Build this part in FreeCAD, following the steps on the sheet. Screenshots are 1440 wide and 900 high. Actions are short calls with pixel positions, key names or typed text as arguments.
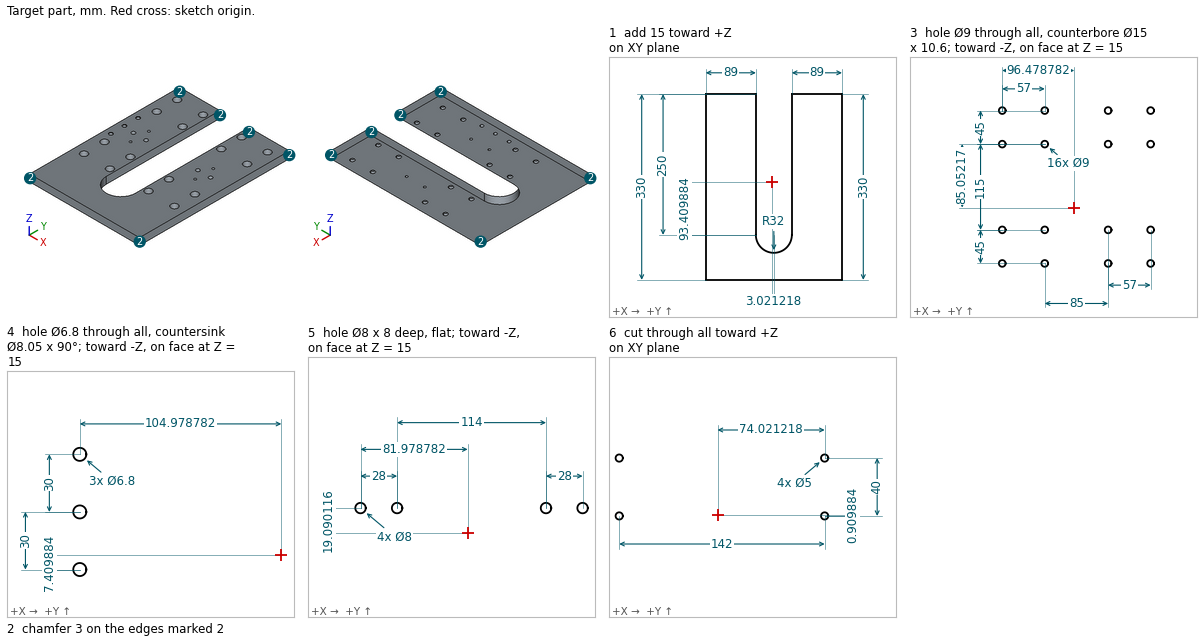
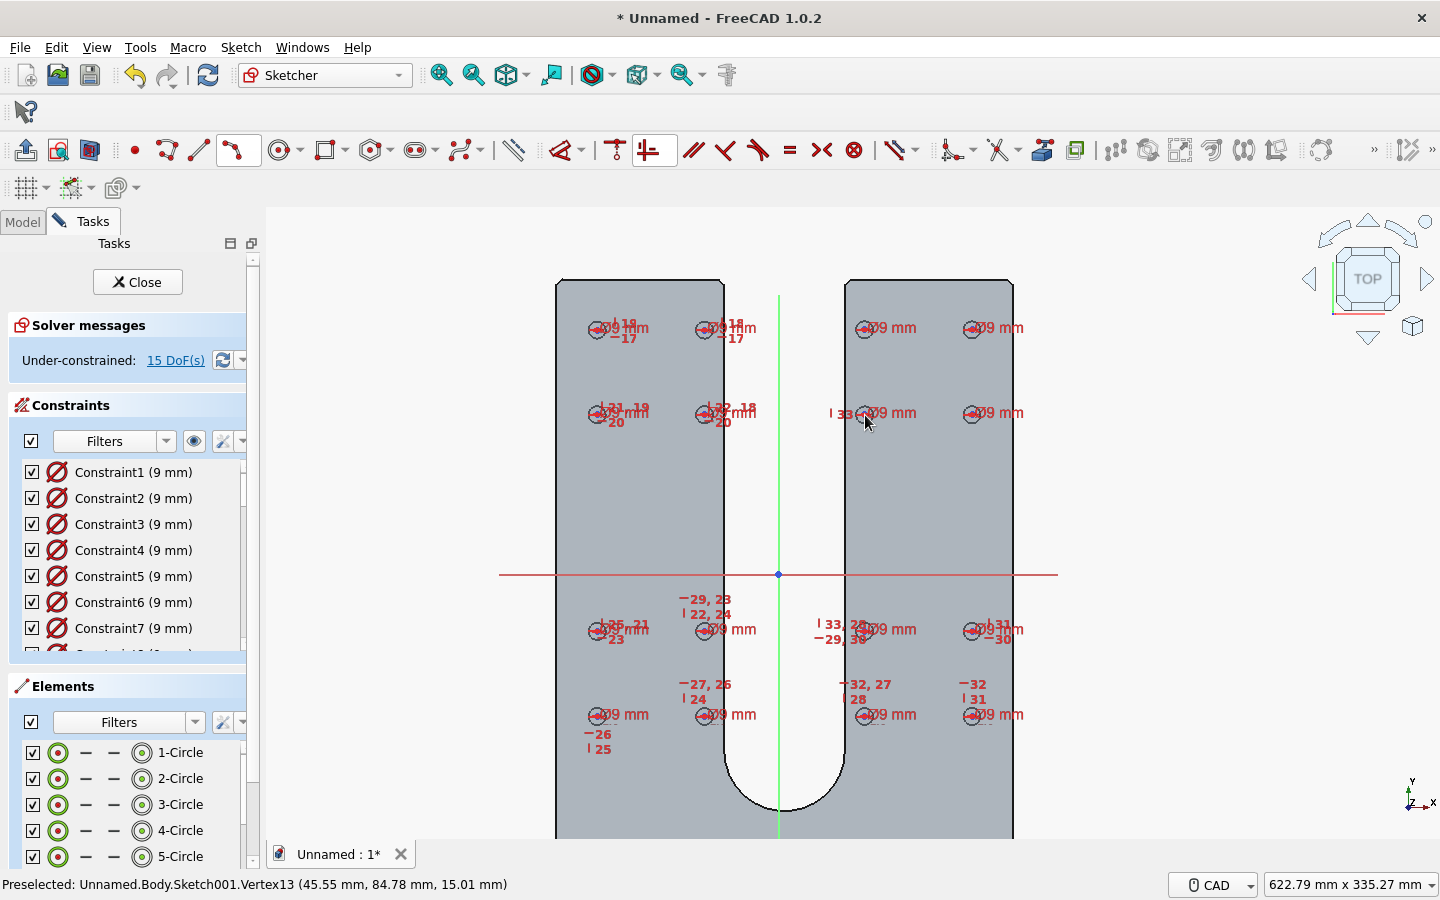
click(705, 415)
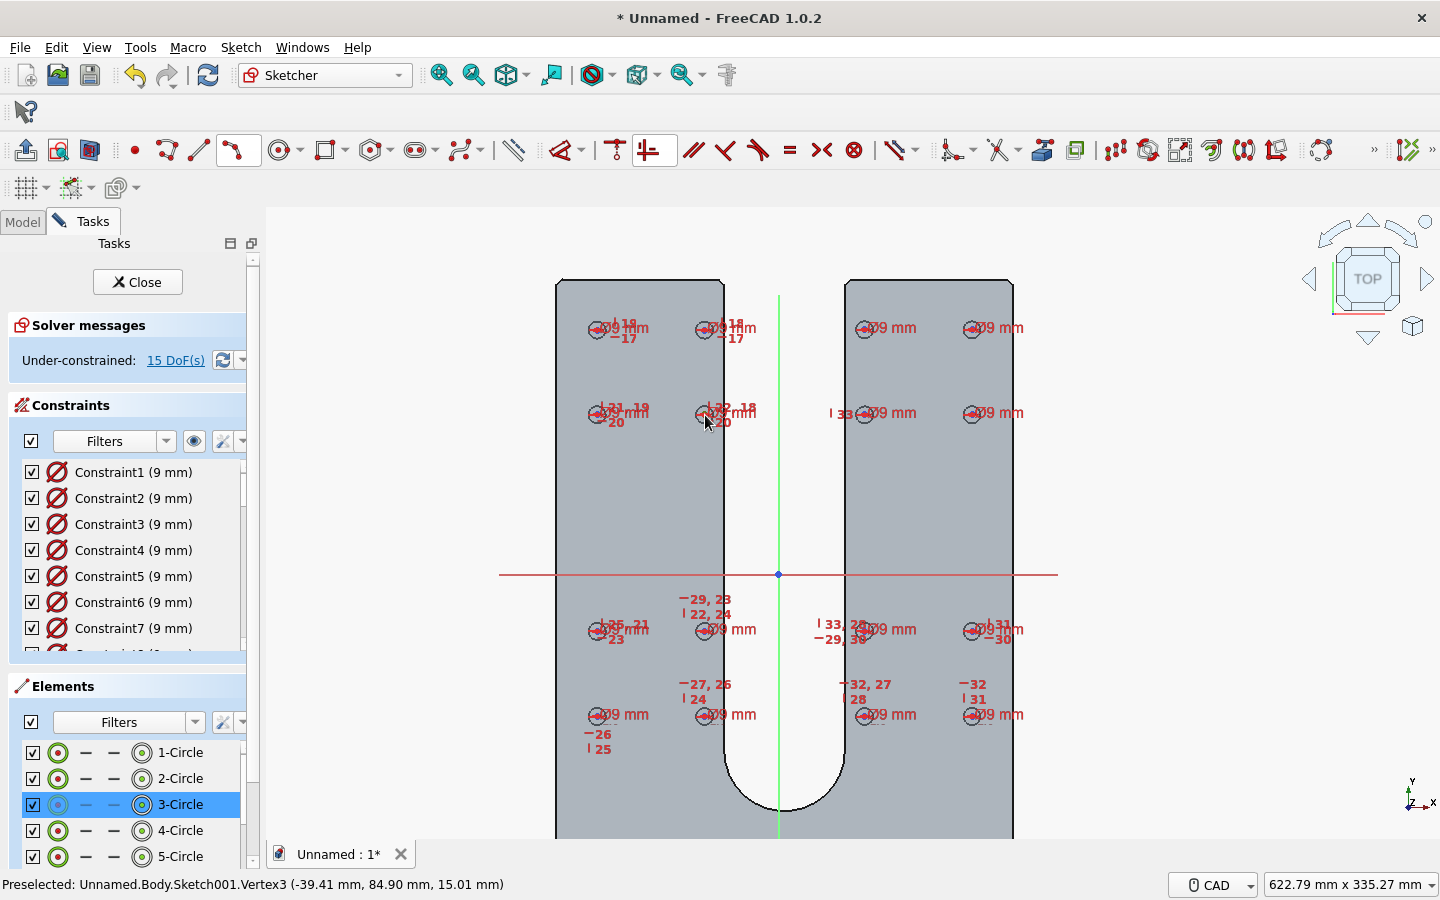
click(865, 415)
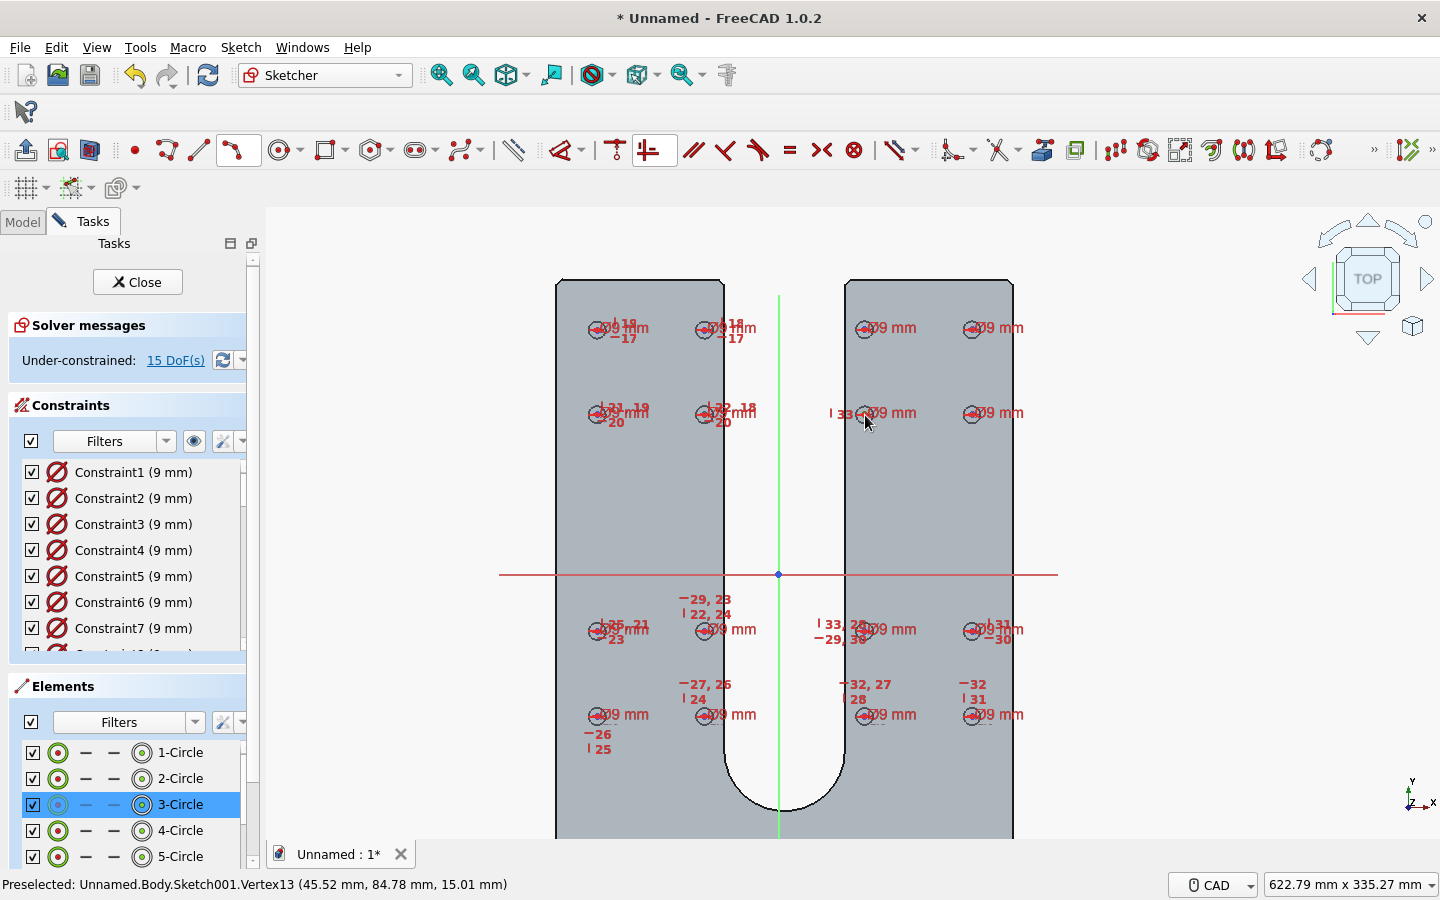
key(h)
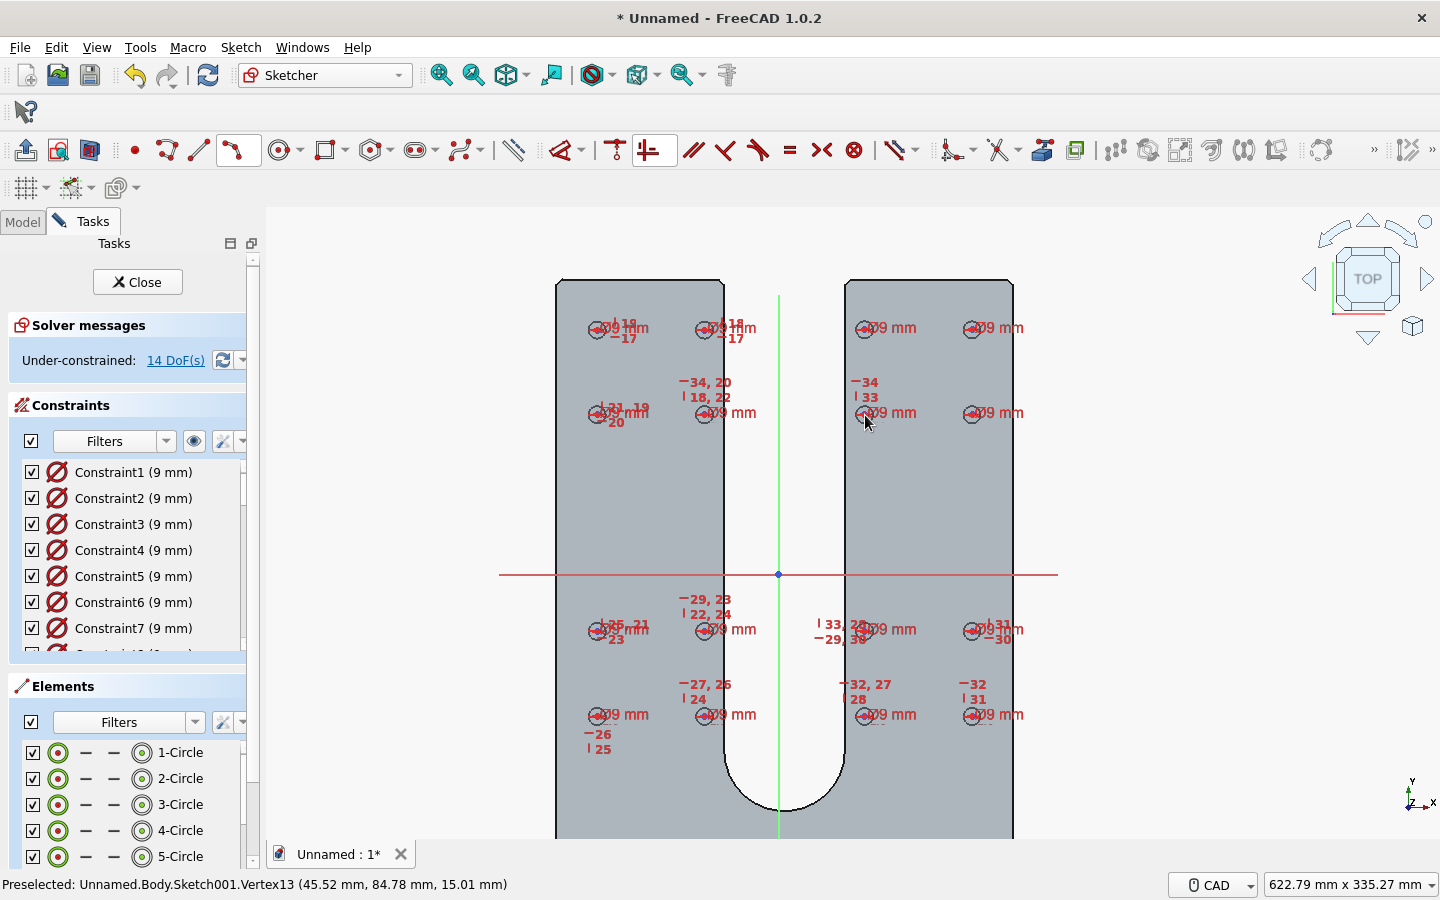
click(865, 415)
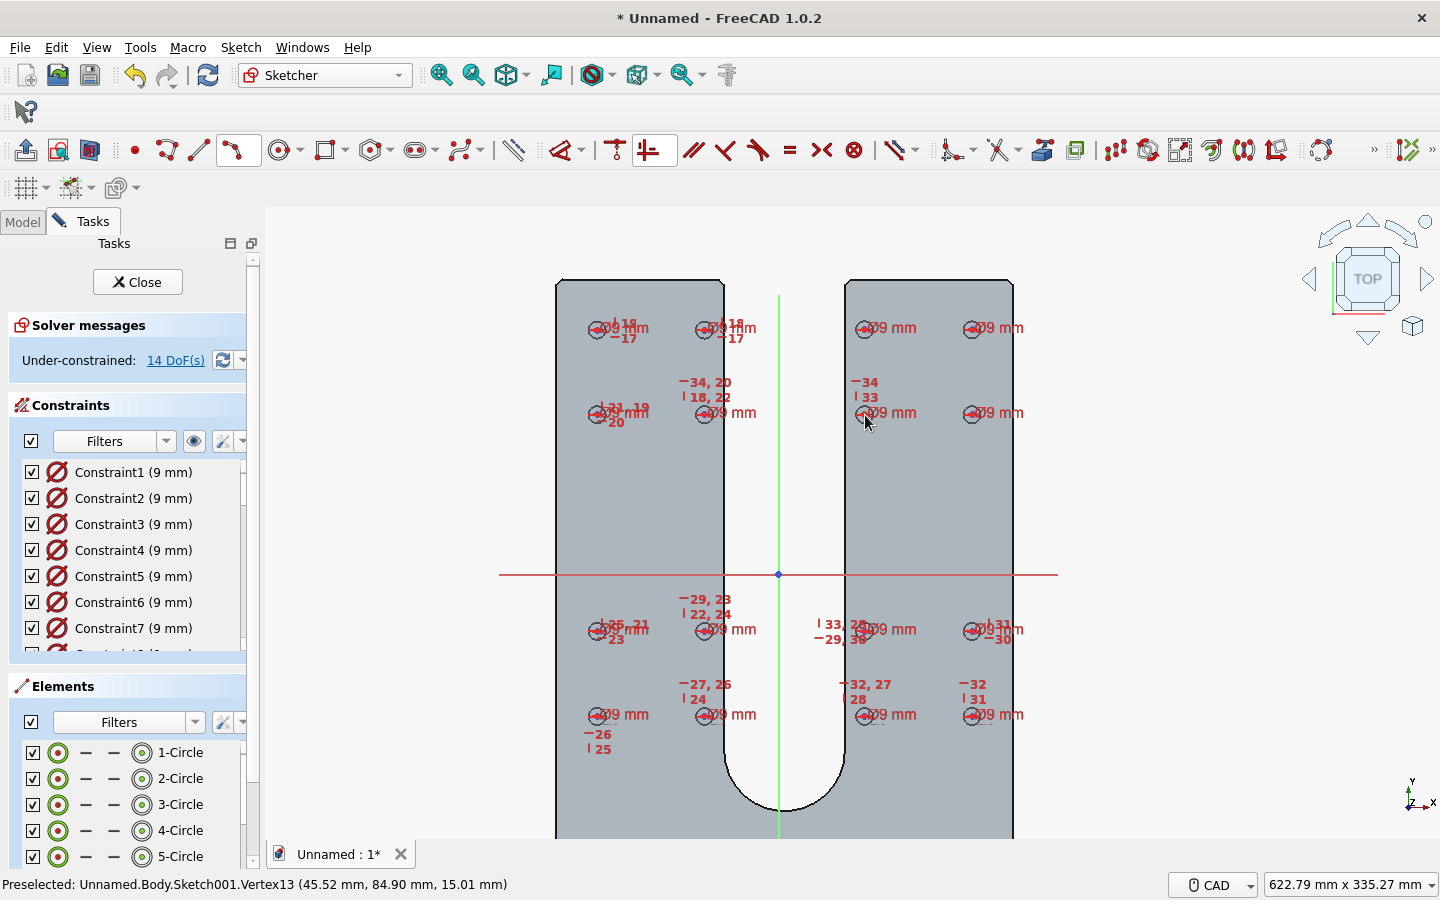
click(865, 330)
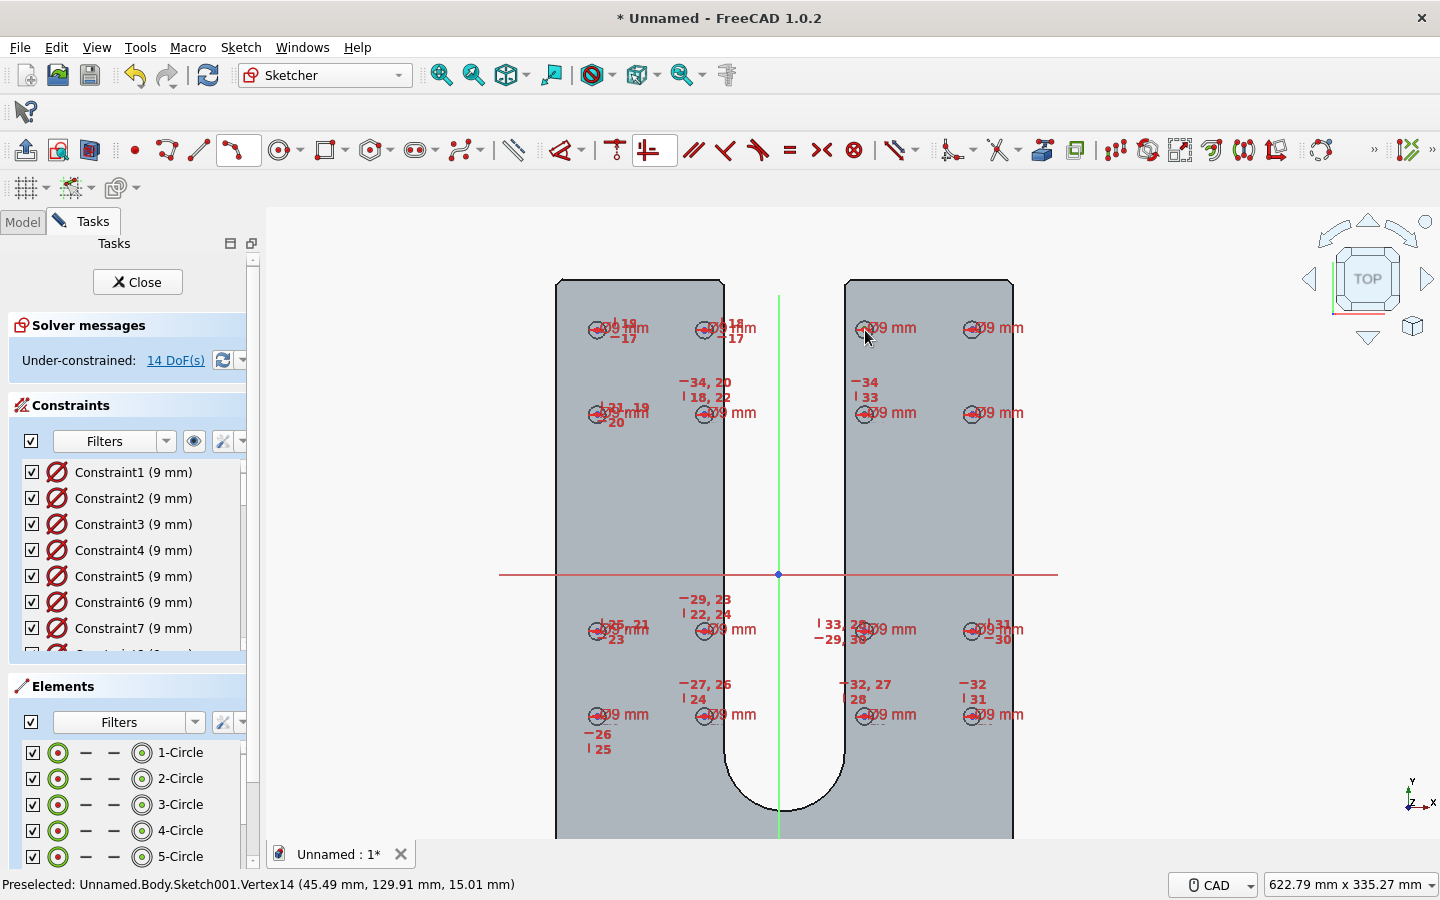
key(v)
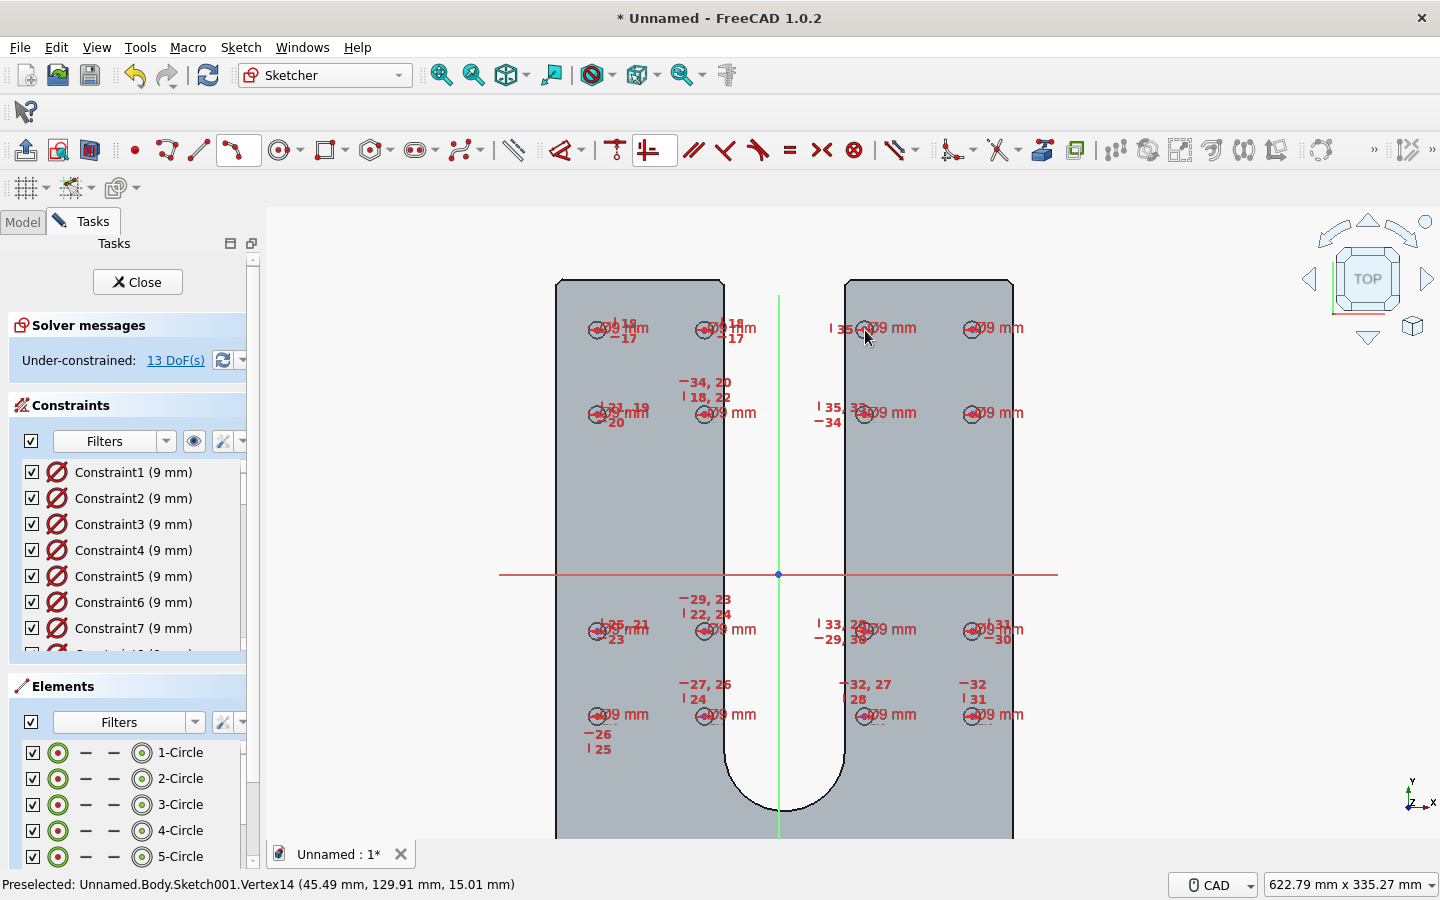
click(705, 330)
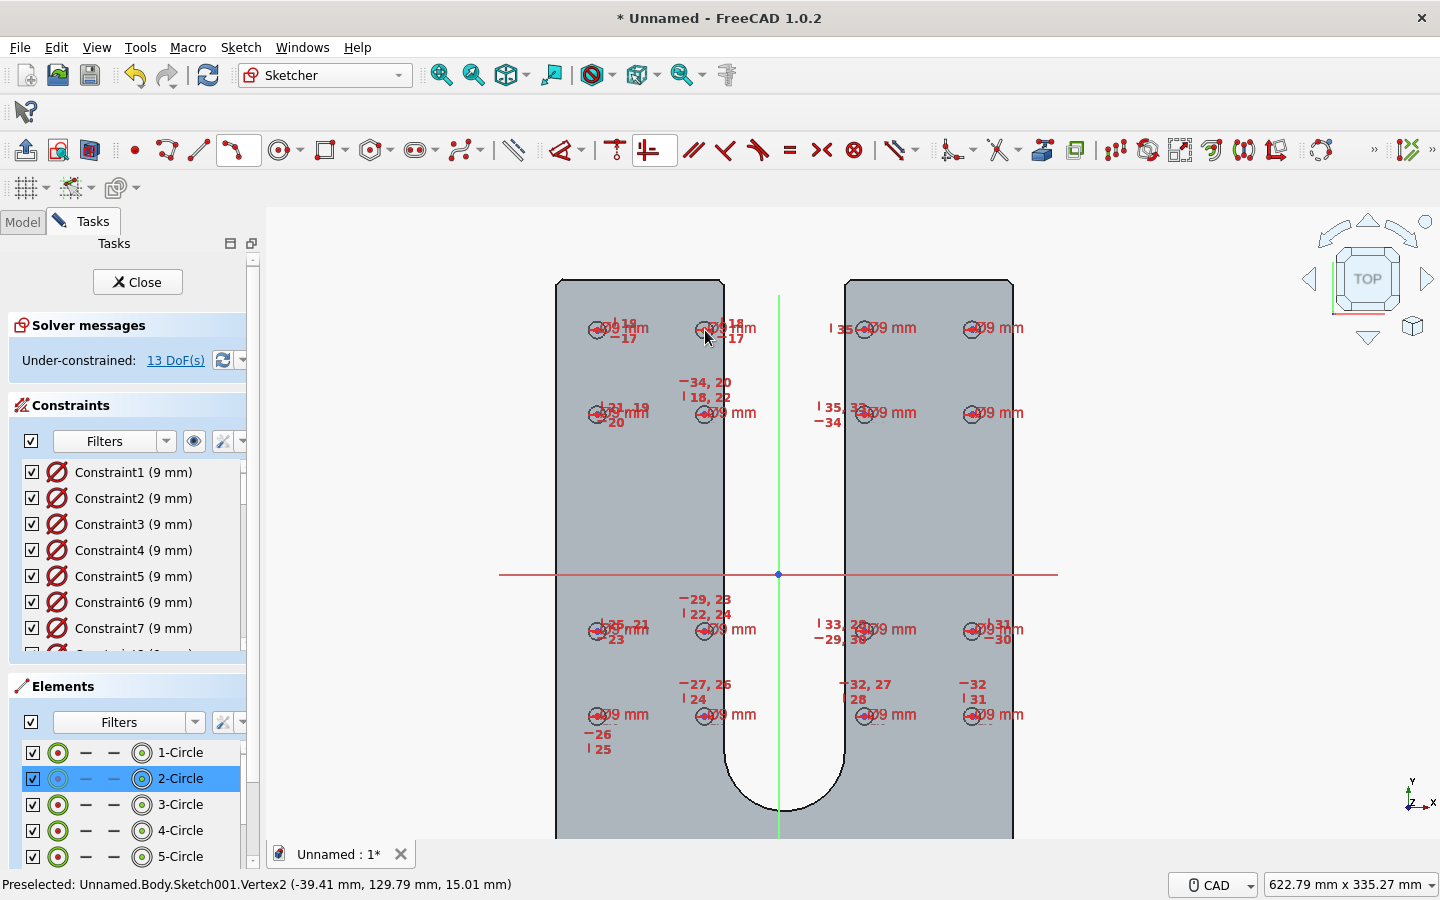
click(865, 330)